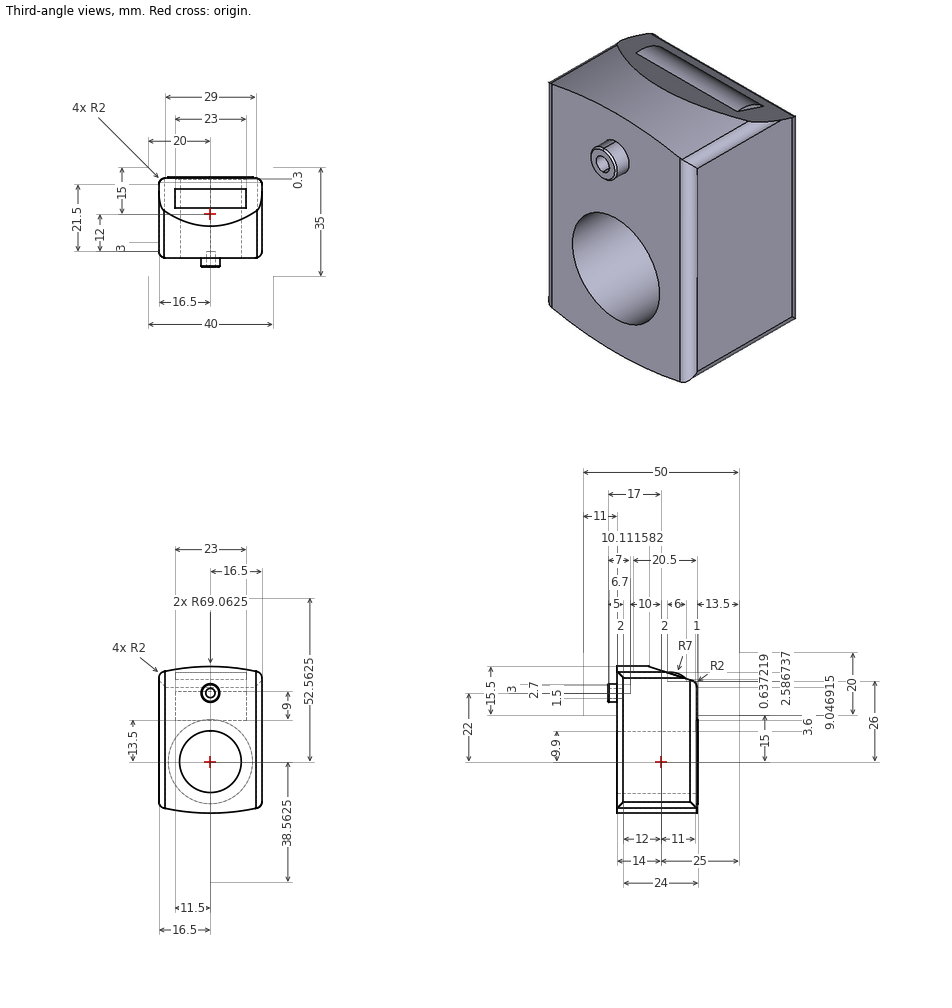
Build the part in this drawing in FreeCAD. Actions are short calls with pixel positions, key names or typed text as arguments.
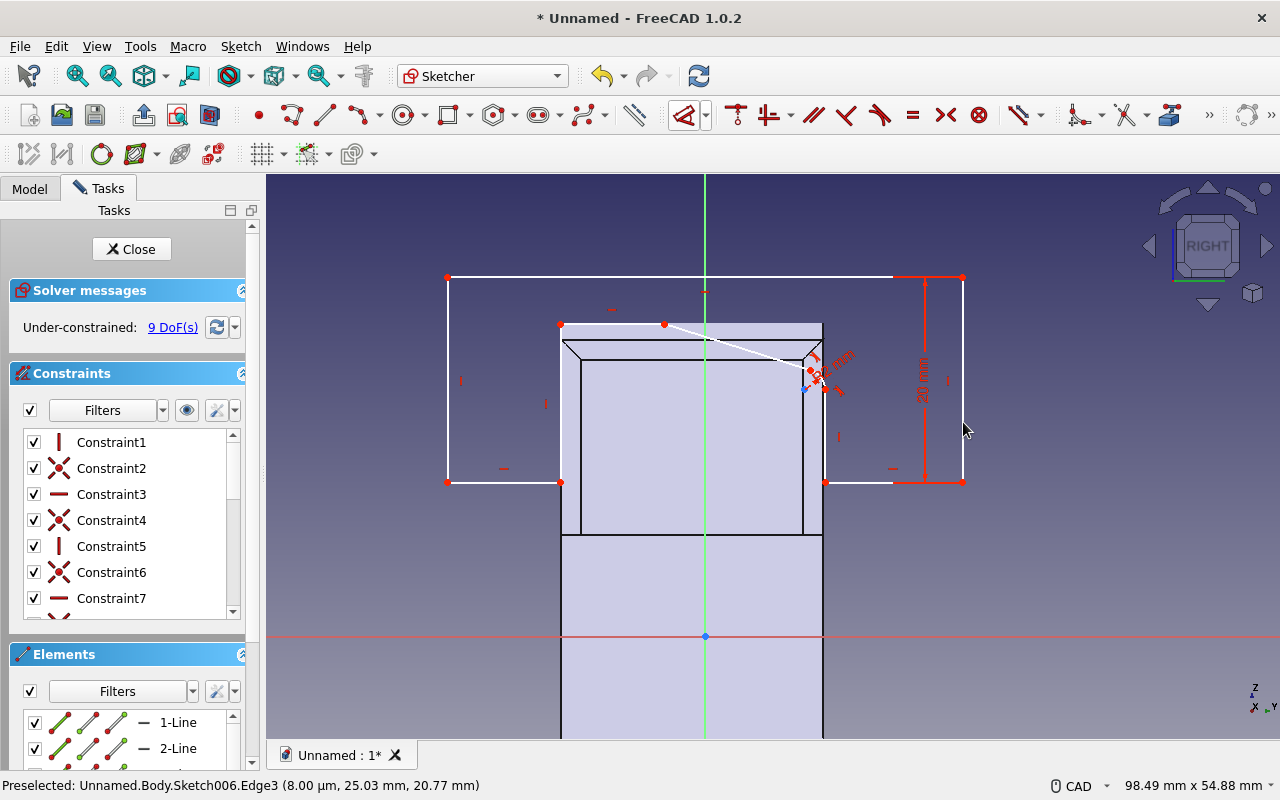
click(808, 277)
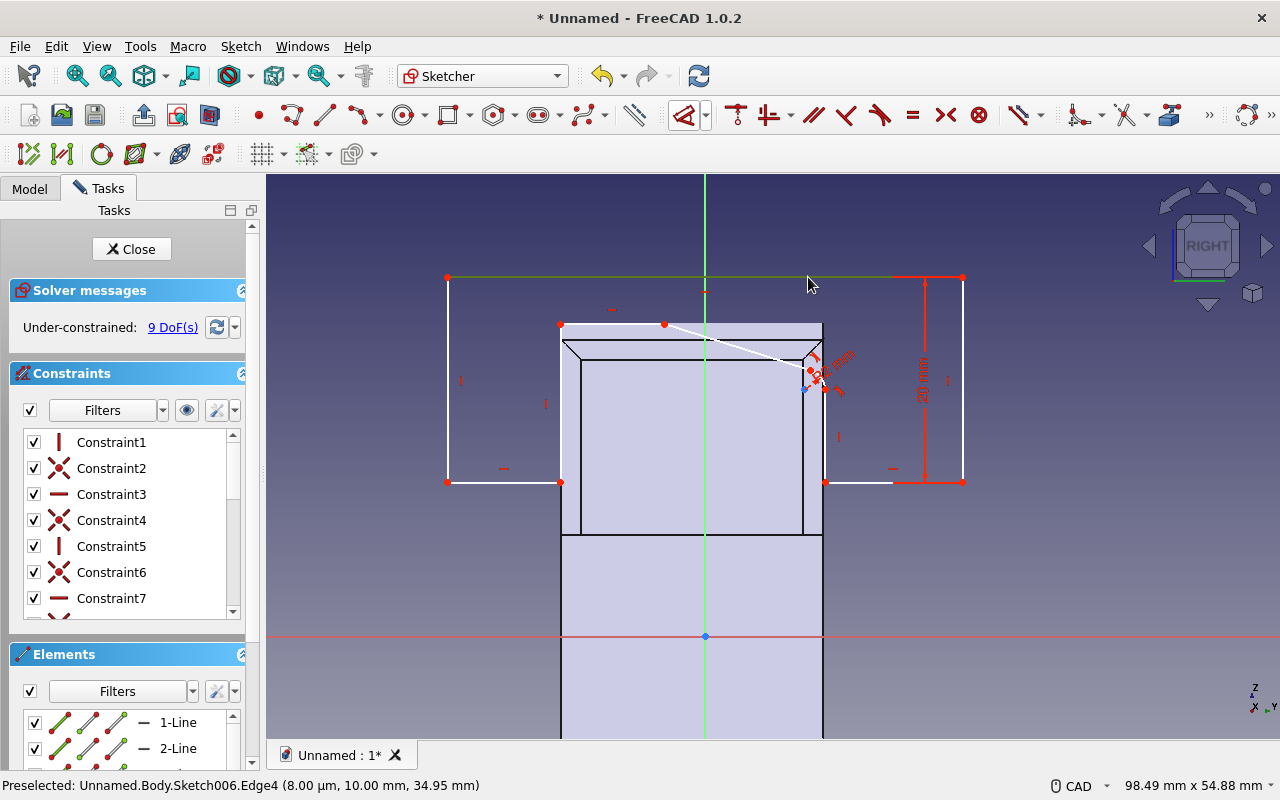
click(706, 116)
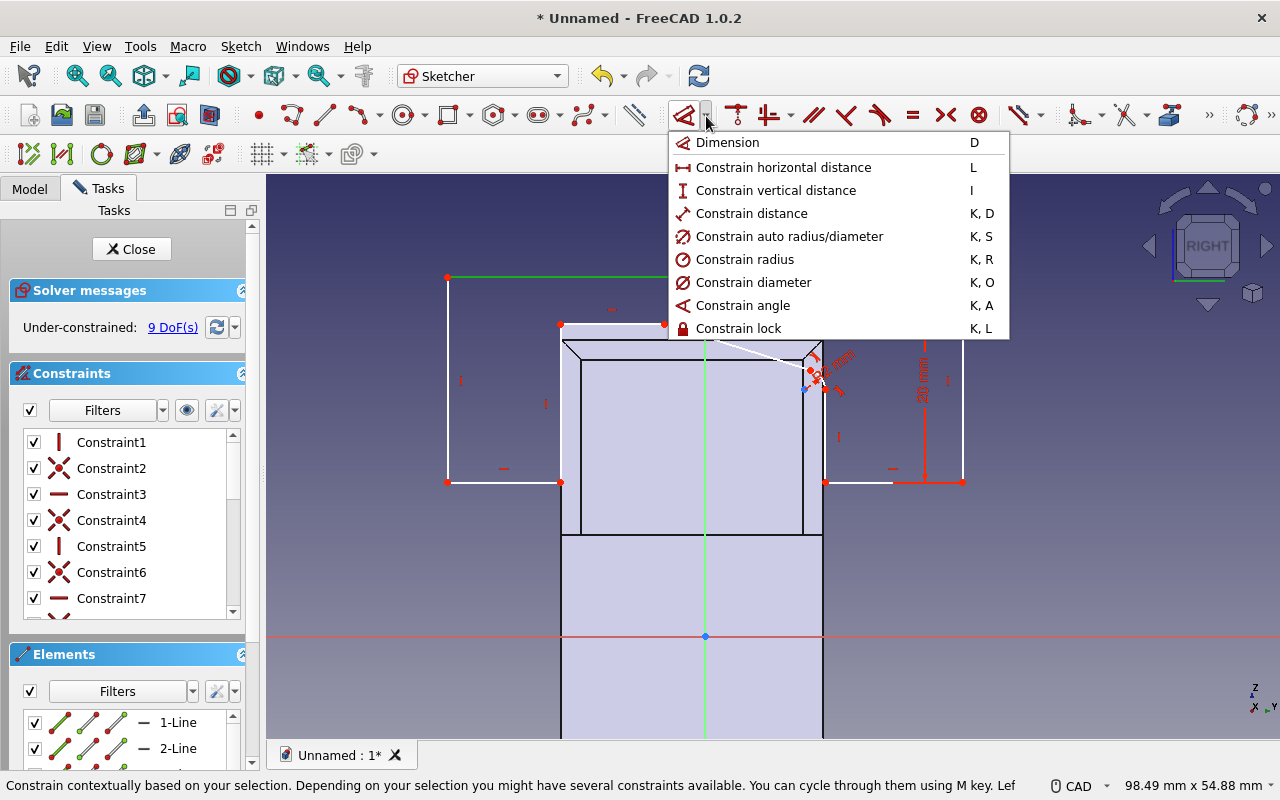
click(839, 168)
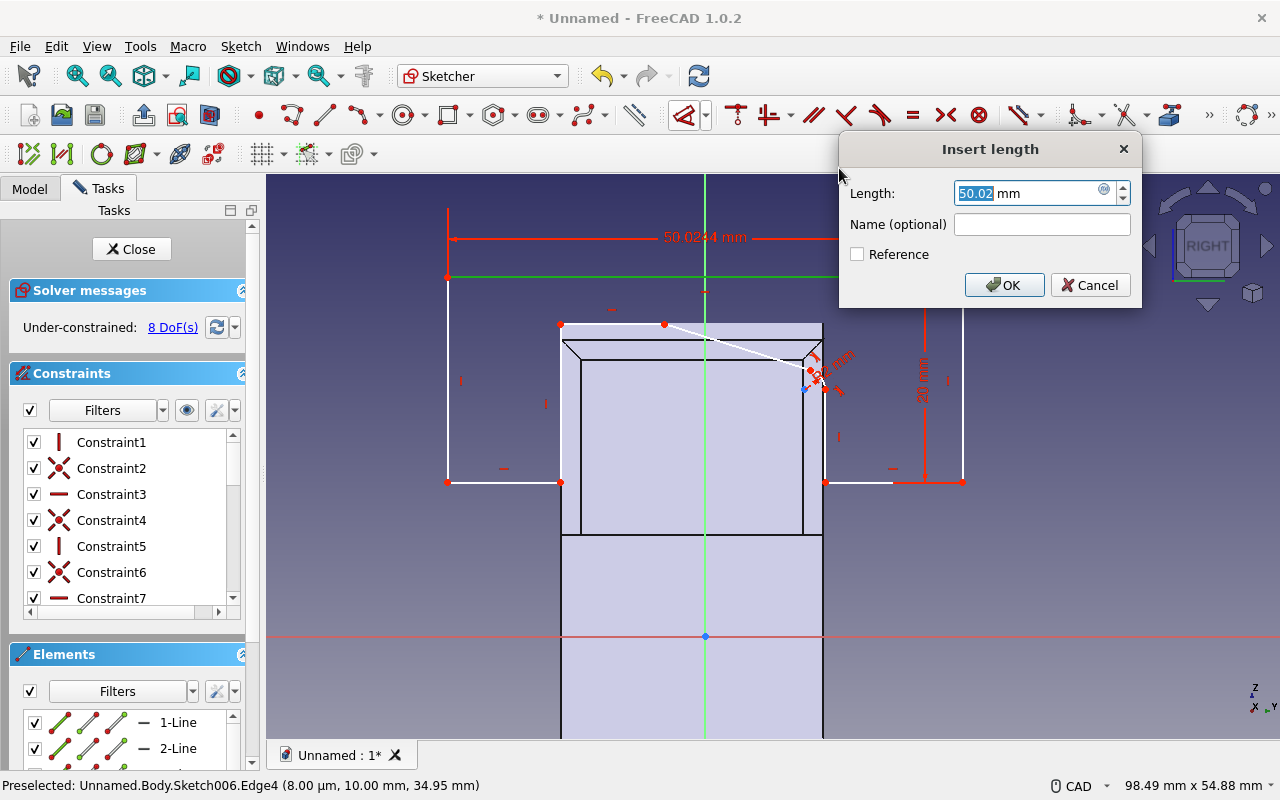
text(50)
key(Return)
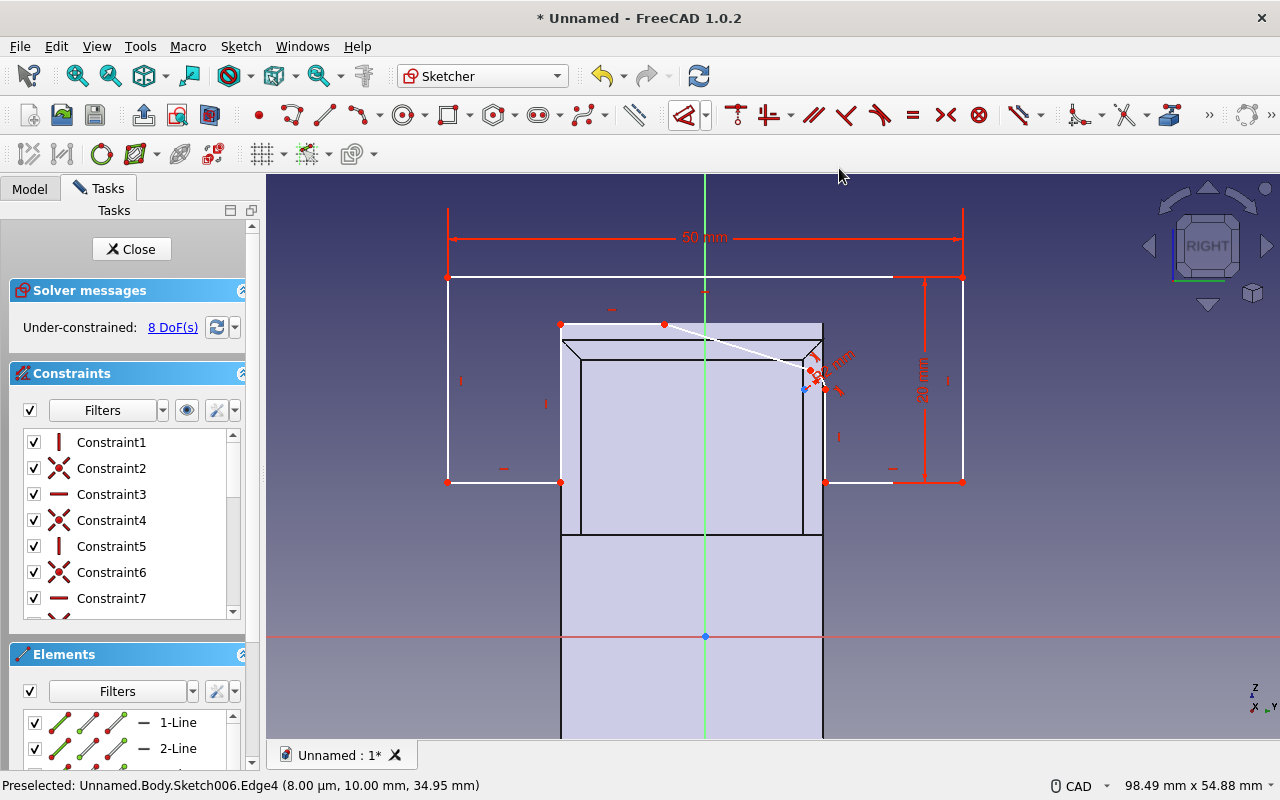
click(448, 339)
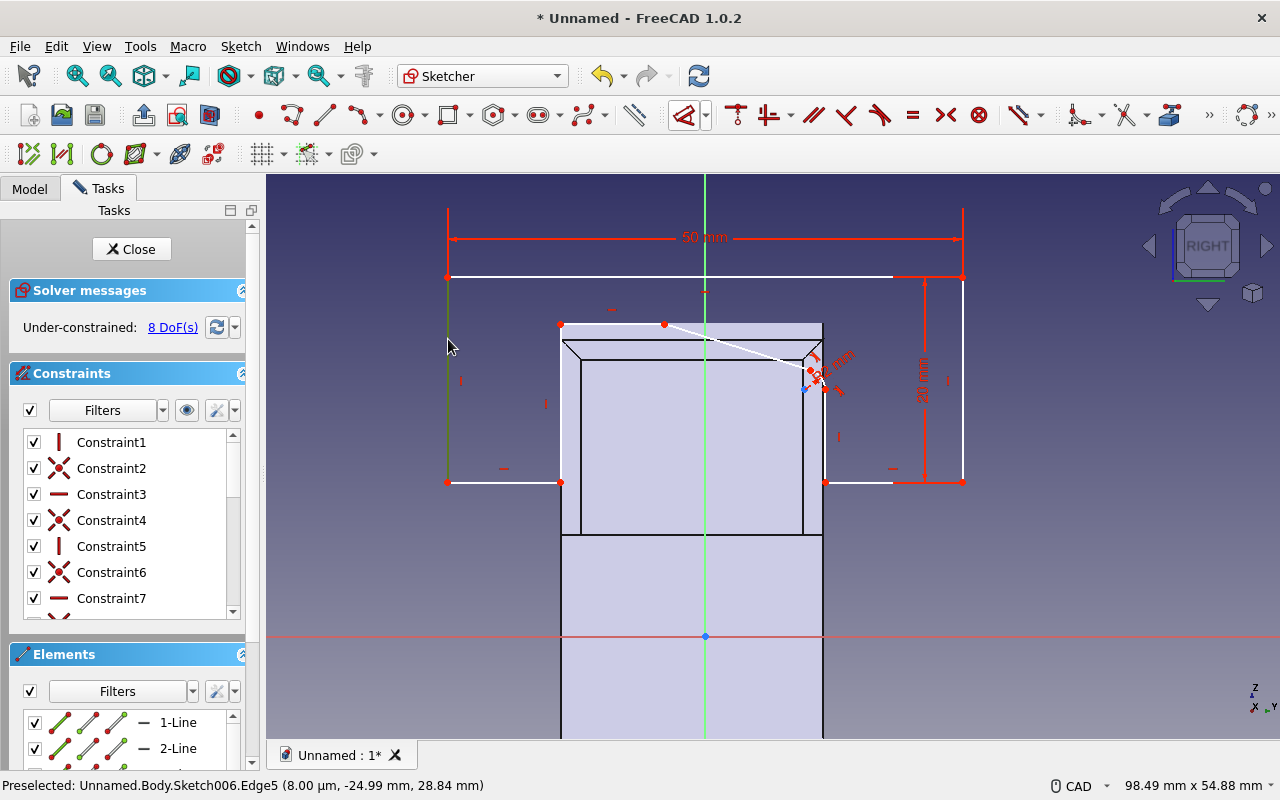
click(706, 116)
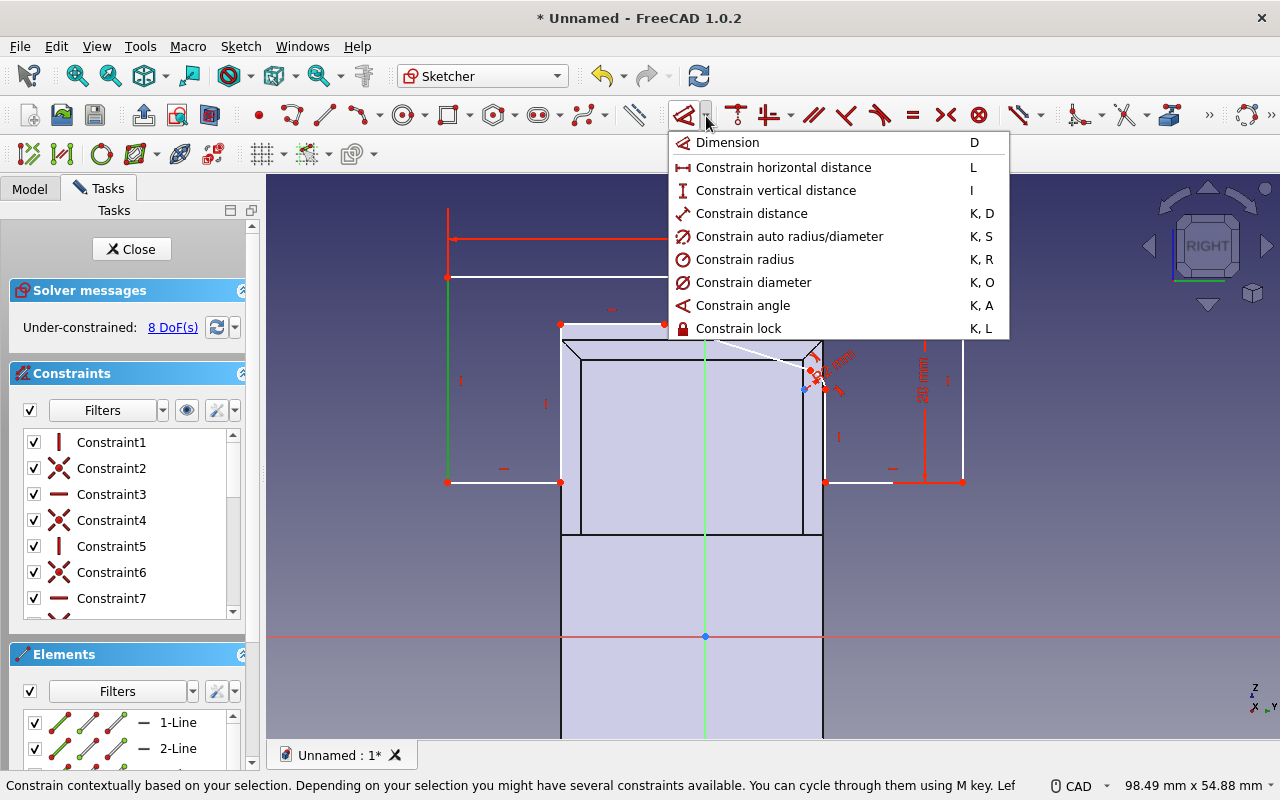
click(839, 190)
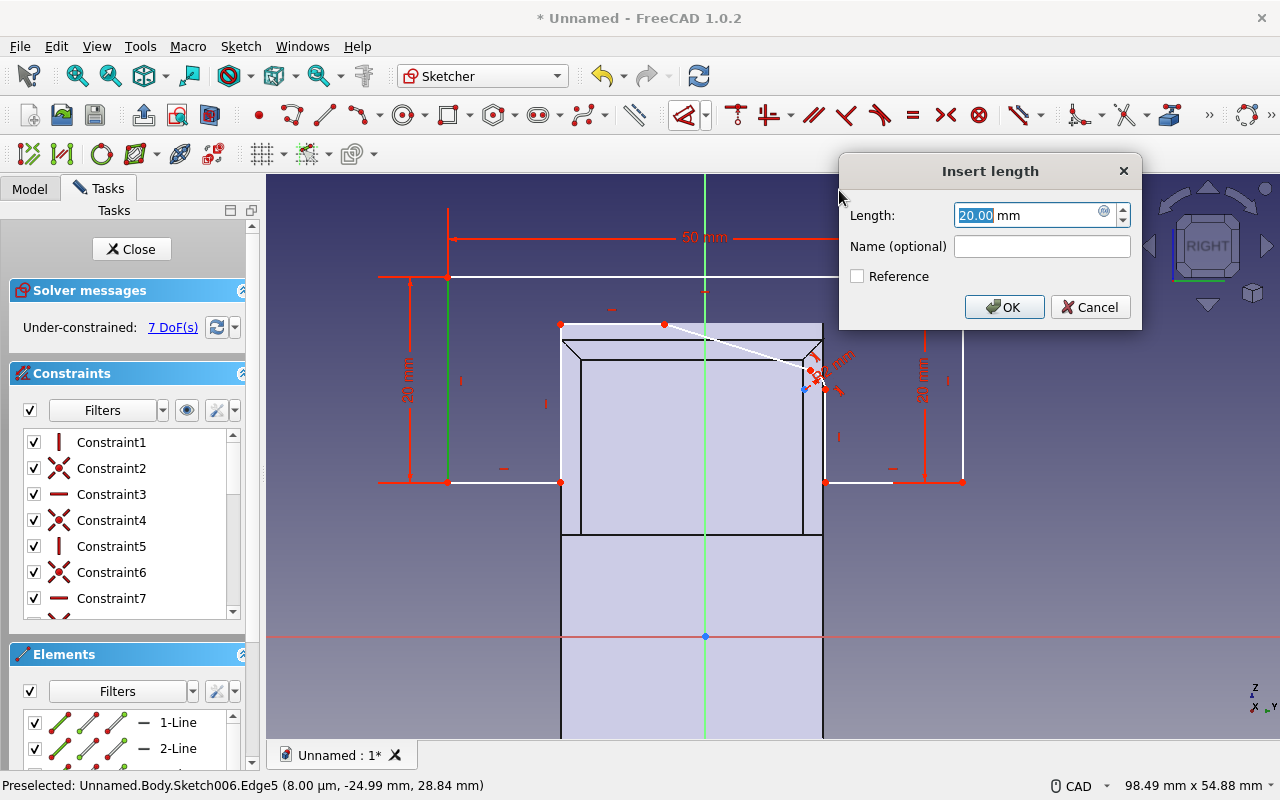
text(20)
key(Return)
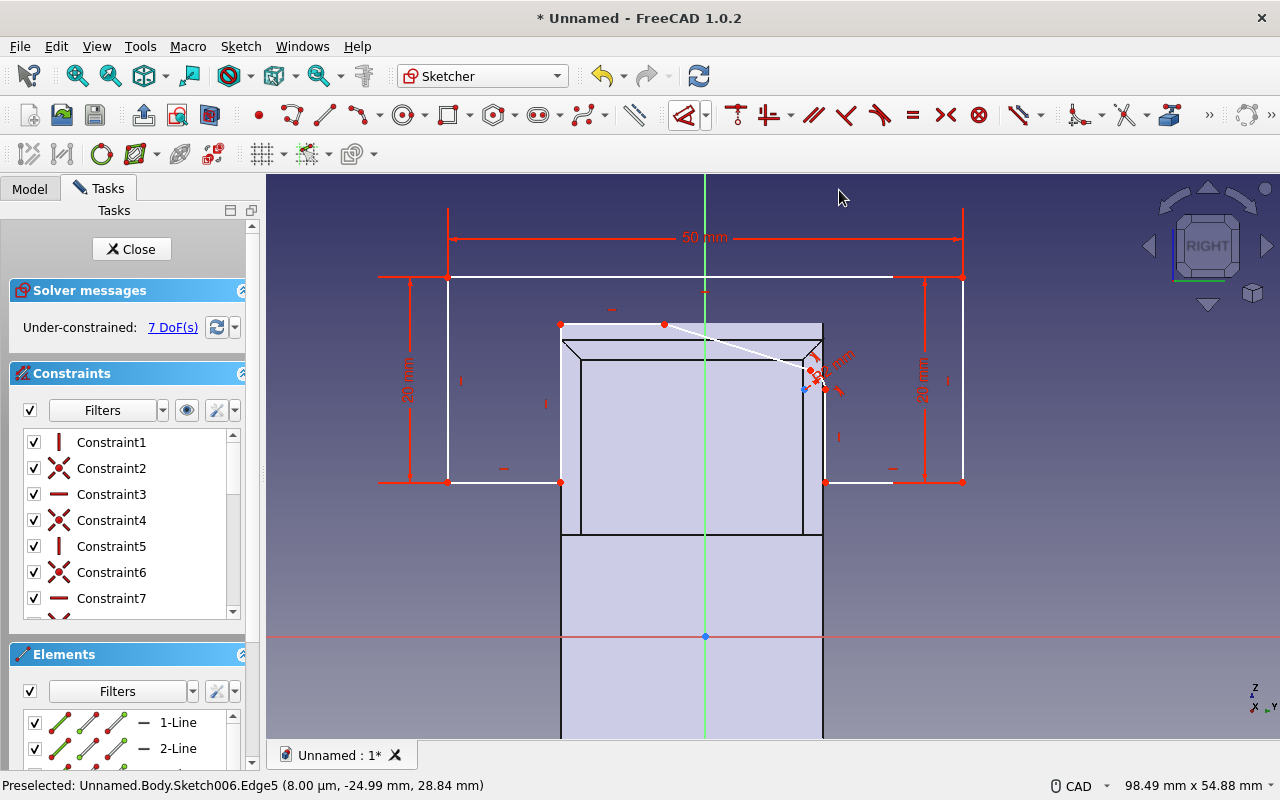
click(482, 483)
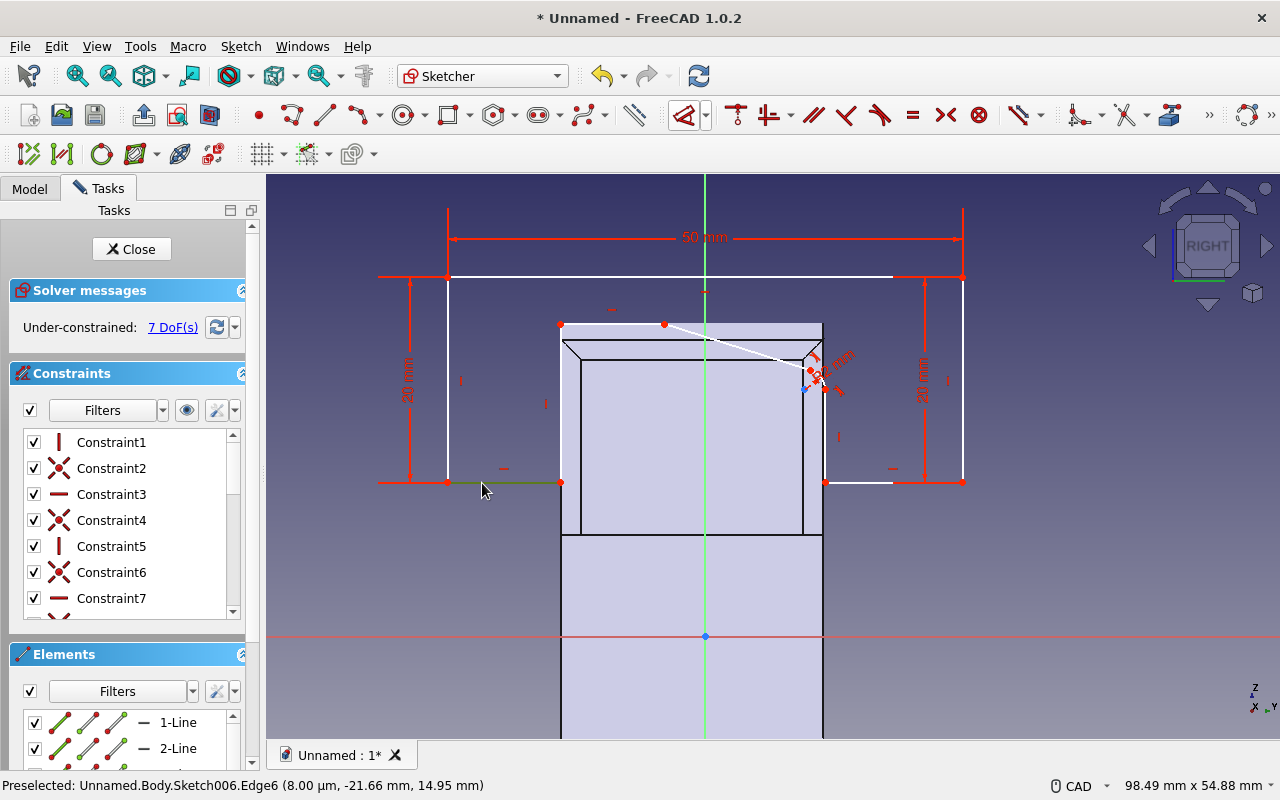
key(l)